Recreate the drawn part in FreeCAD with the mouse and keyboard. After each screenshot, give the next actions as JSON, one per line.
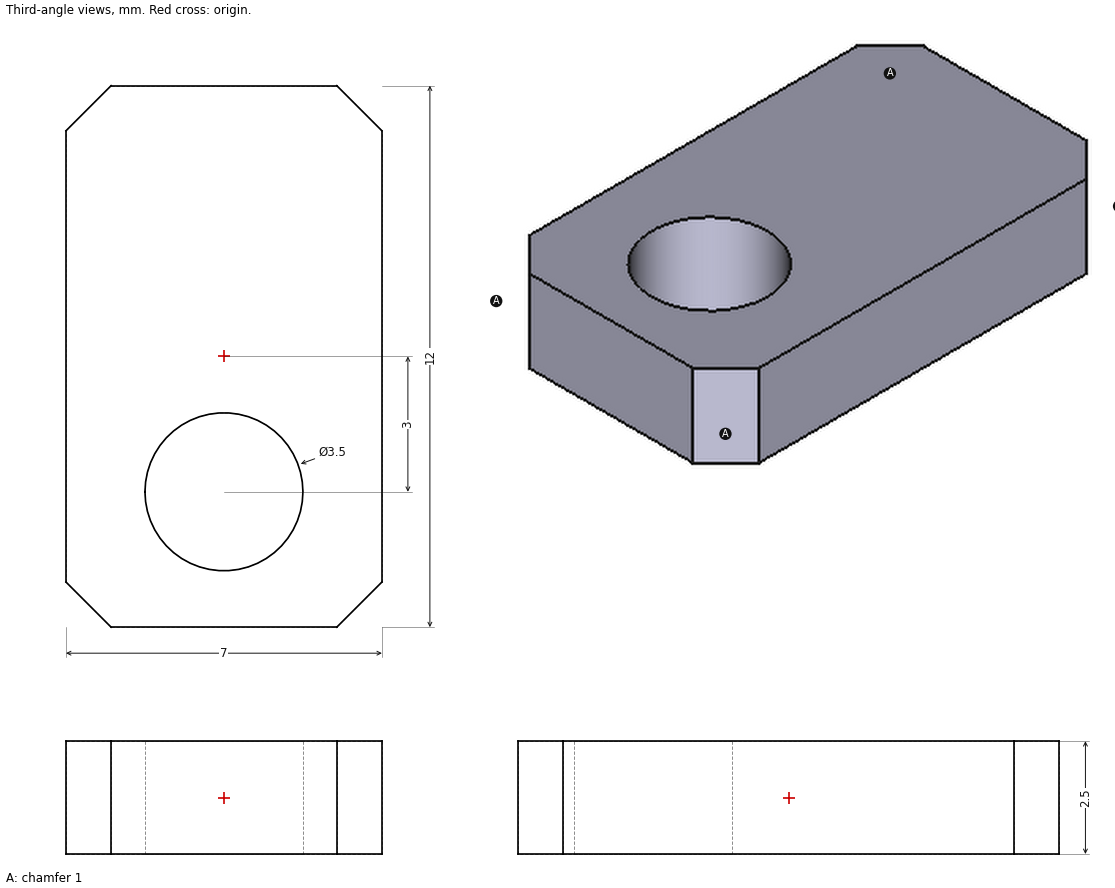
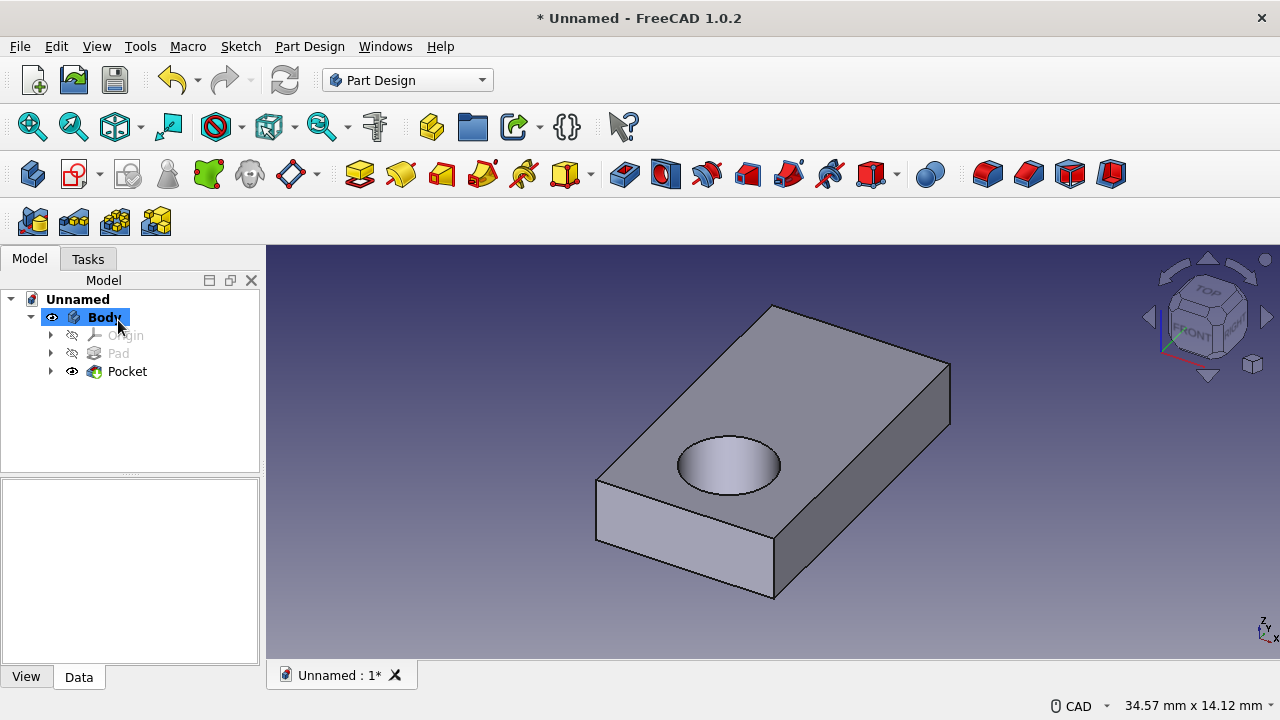
{"action": "left_click", "coordinate": [774, 568]}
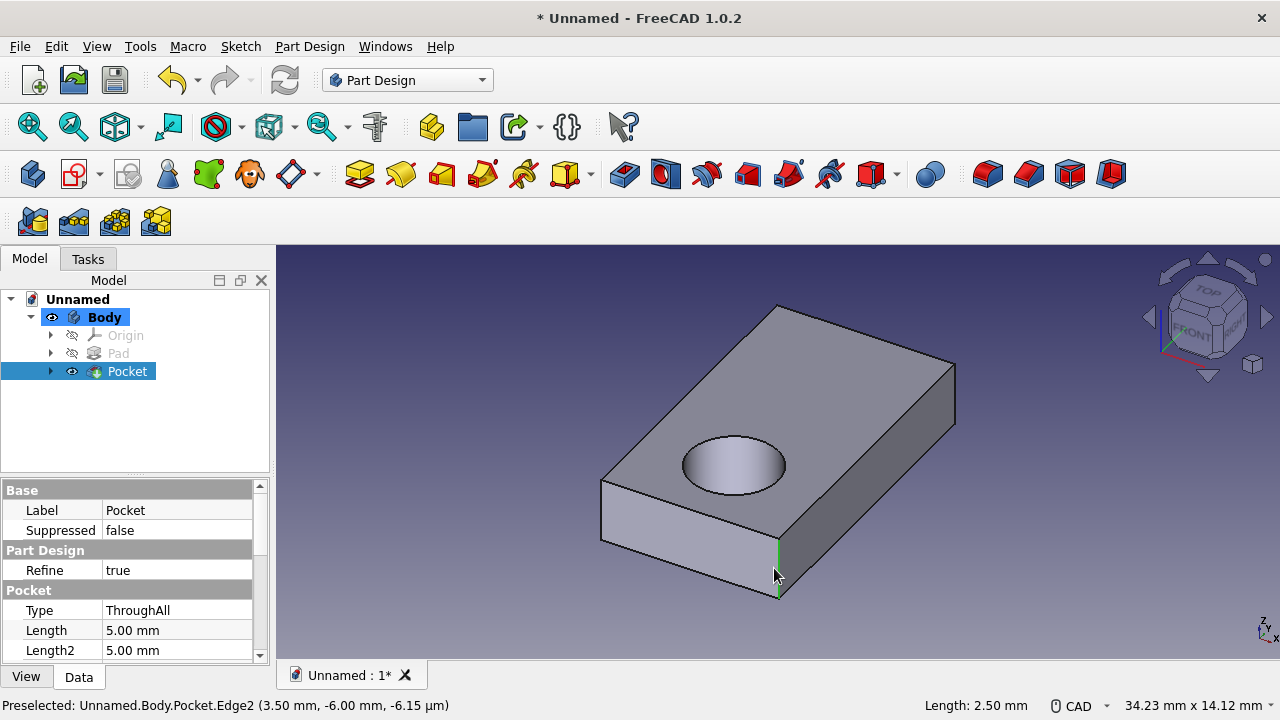
{"action": "key", "text": "0"}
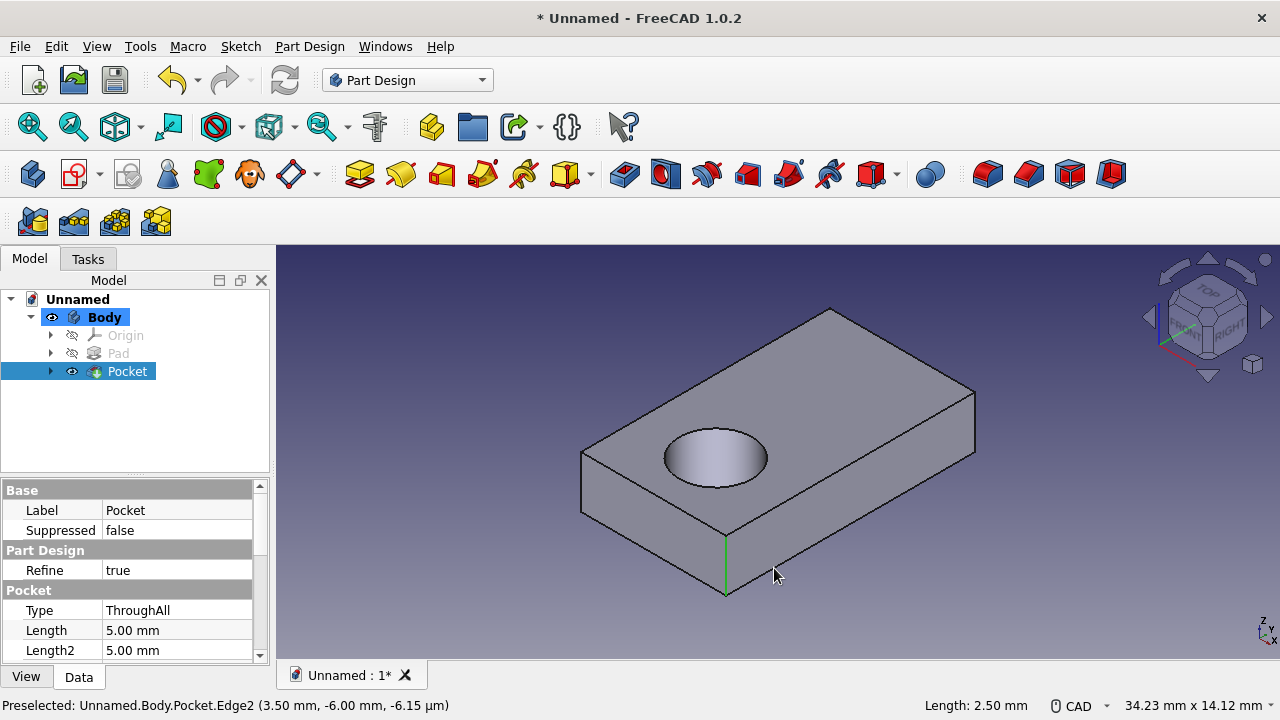
{"action": "key", "text": "2"}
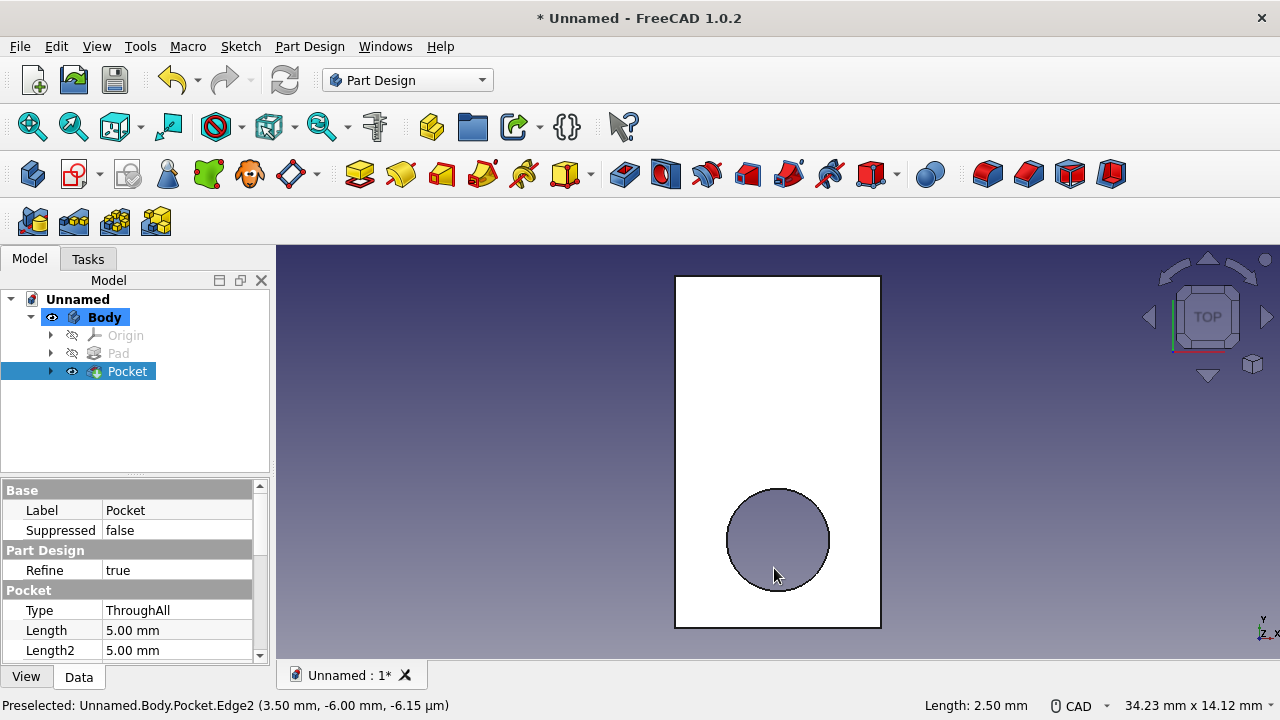
{"action": "key", "text": "1"}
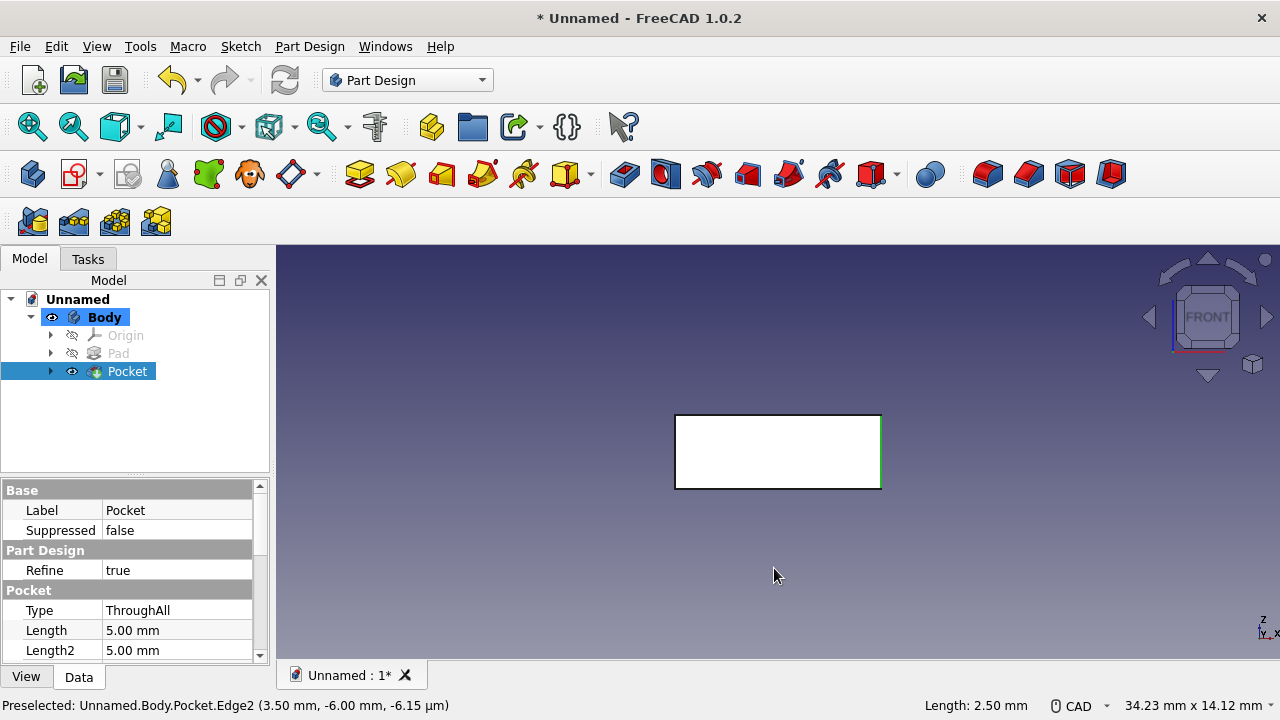
{"action": "left_click", "coordinate": [33, 128]}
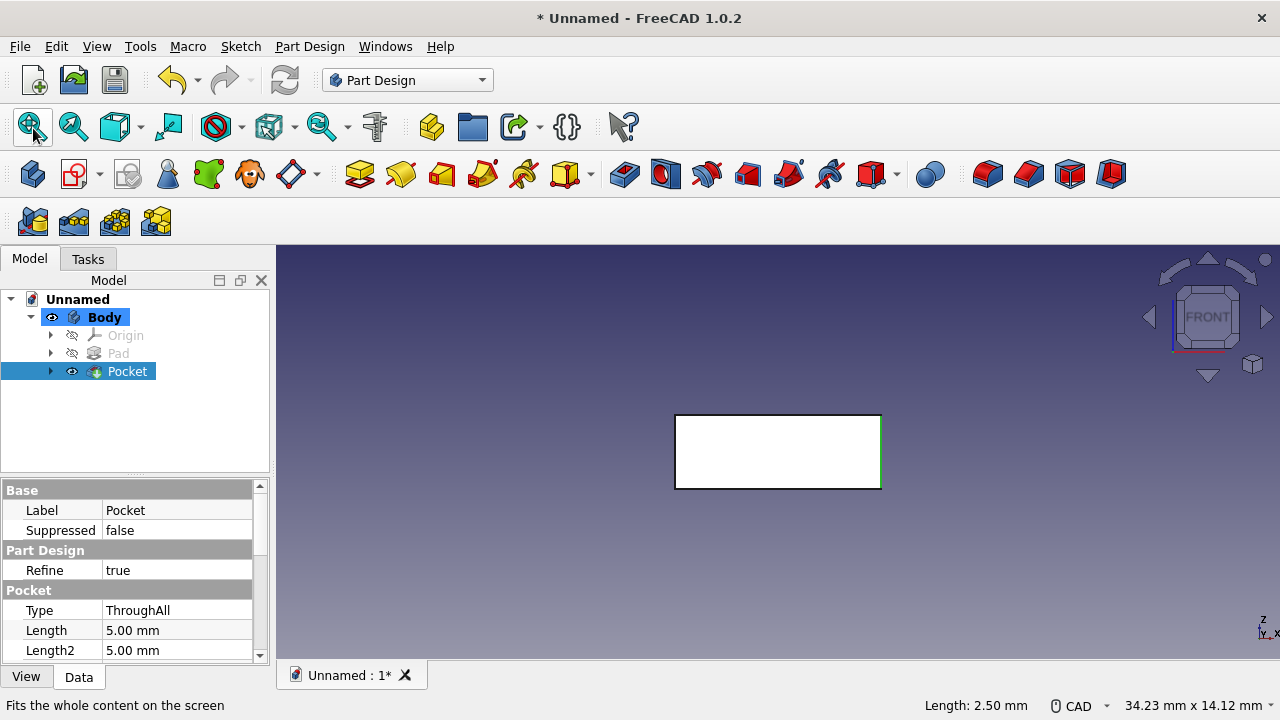
{"action": "left_click", "coordinate": [675, 451], "text": "ctrl"}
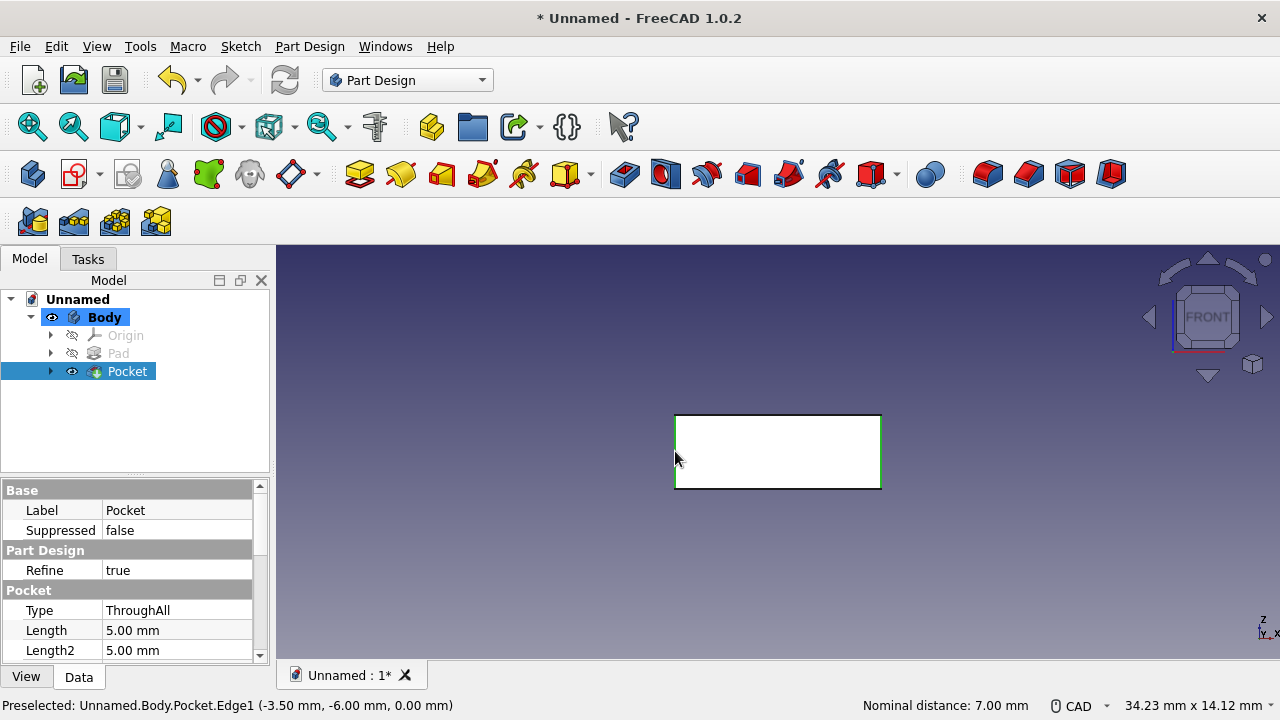
{"action": "key", "text": "3"}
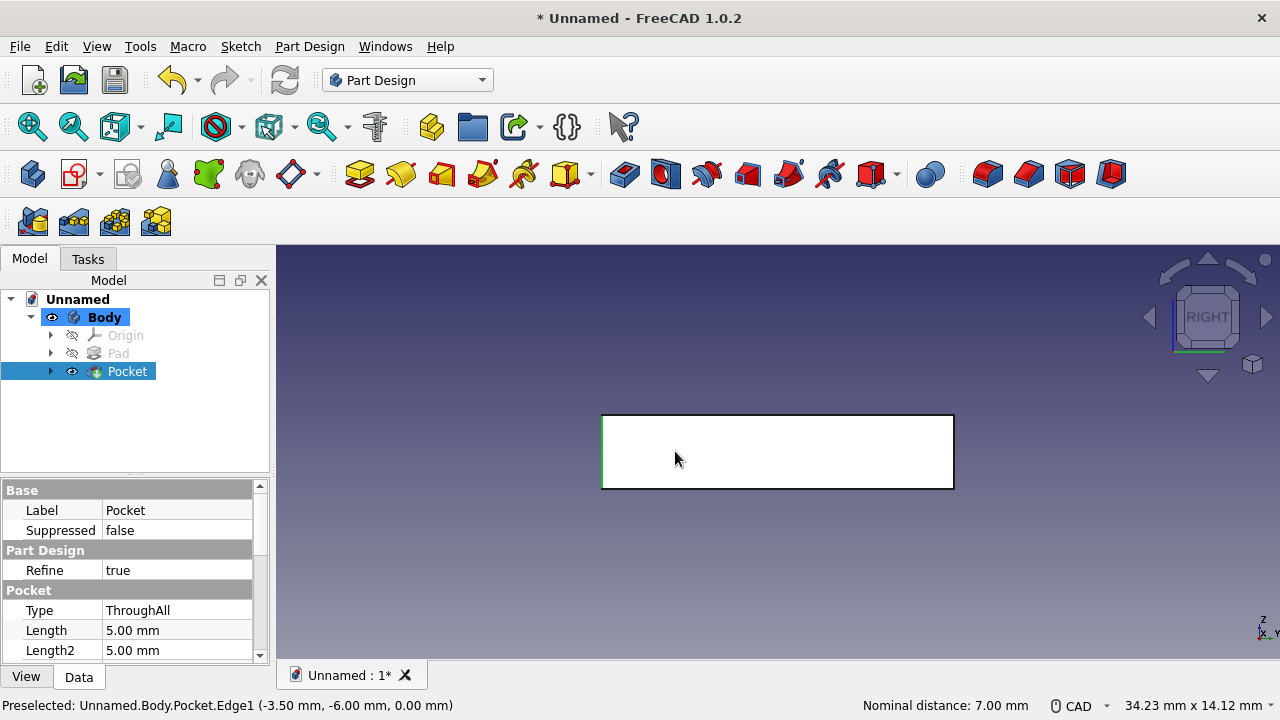
{"action": "left_click", "coordinate": [33, 128]}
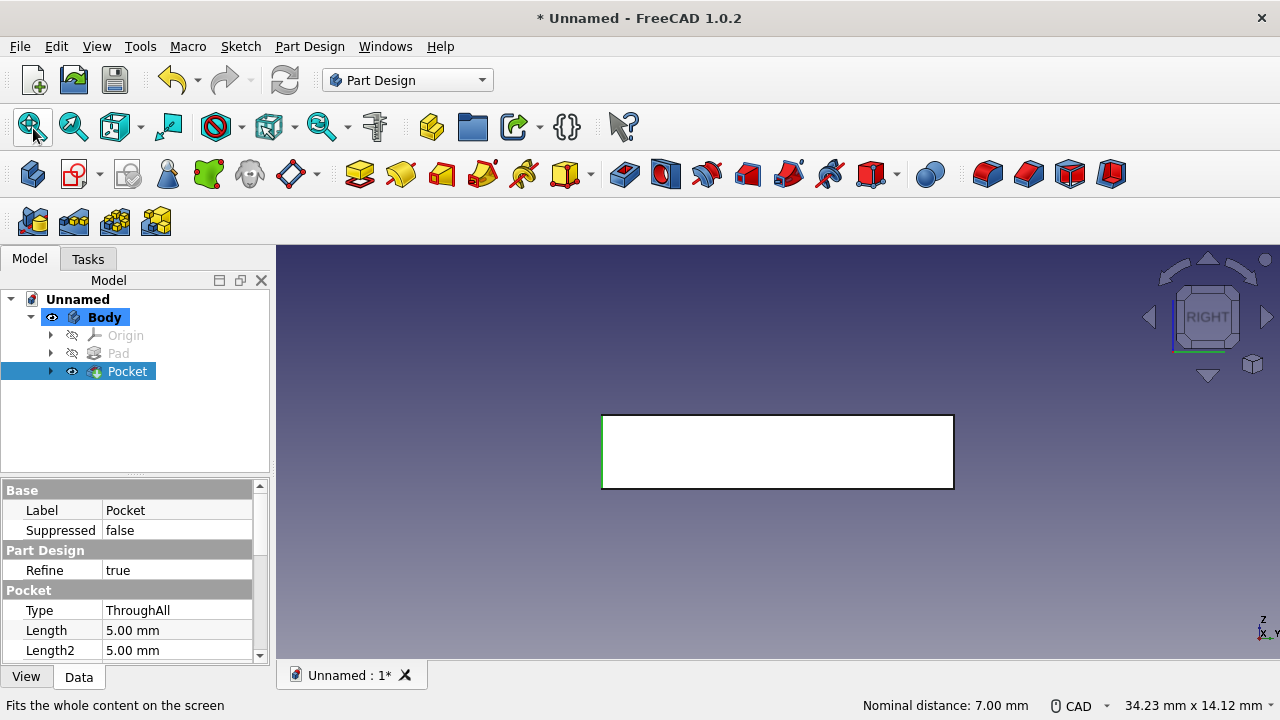
{"action": "left_click", "coordinate": [954, 451], "text": "ctrl"}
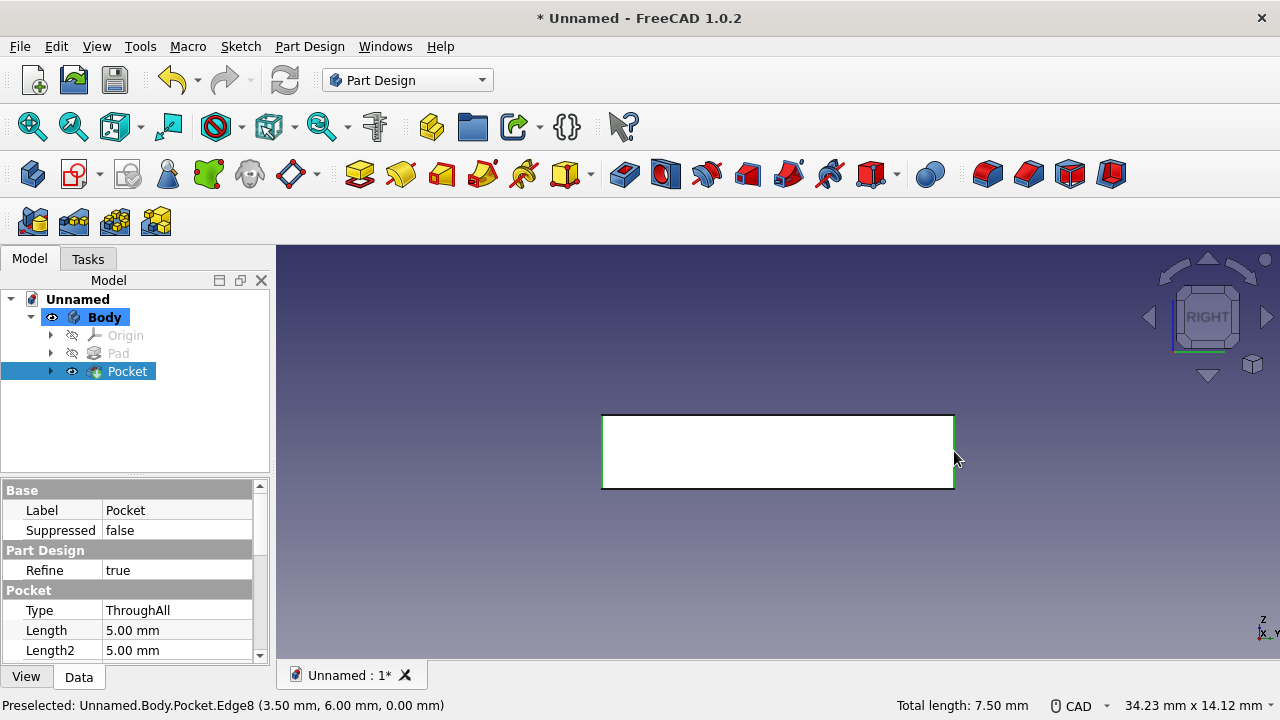
{"action": "key", "text": "5"}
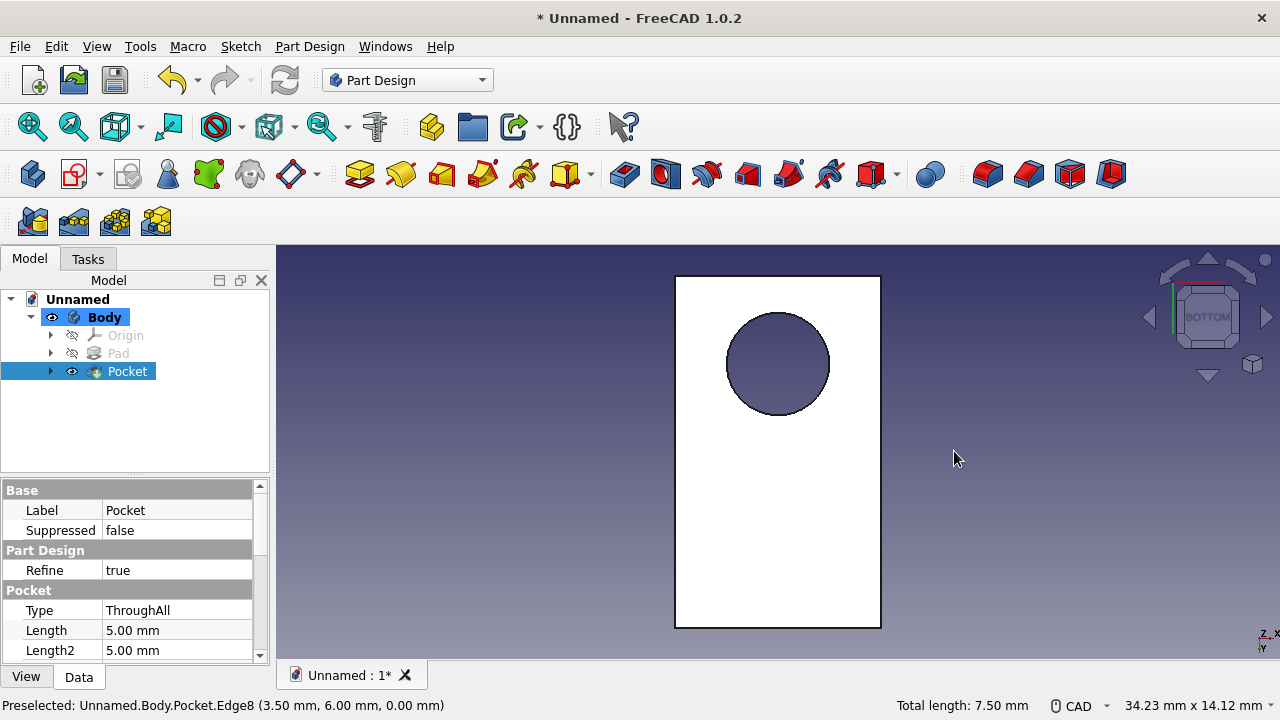
{"action": "key", "text": "4"}